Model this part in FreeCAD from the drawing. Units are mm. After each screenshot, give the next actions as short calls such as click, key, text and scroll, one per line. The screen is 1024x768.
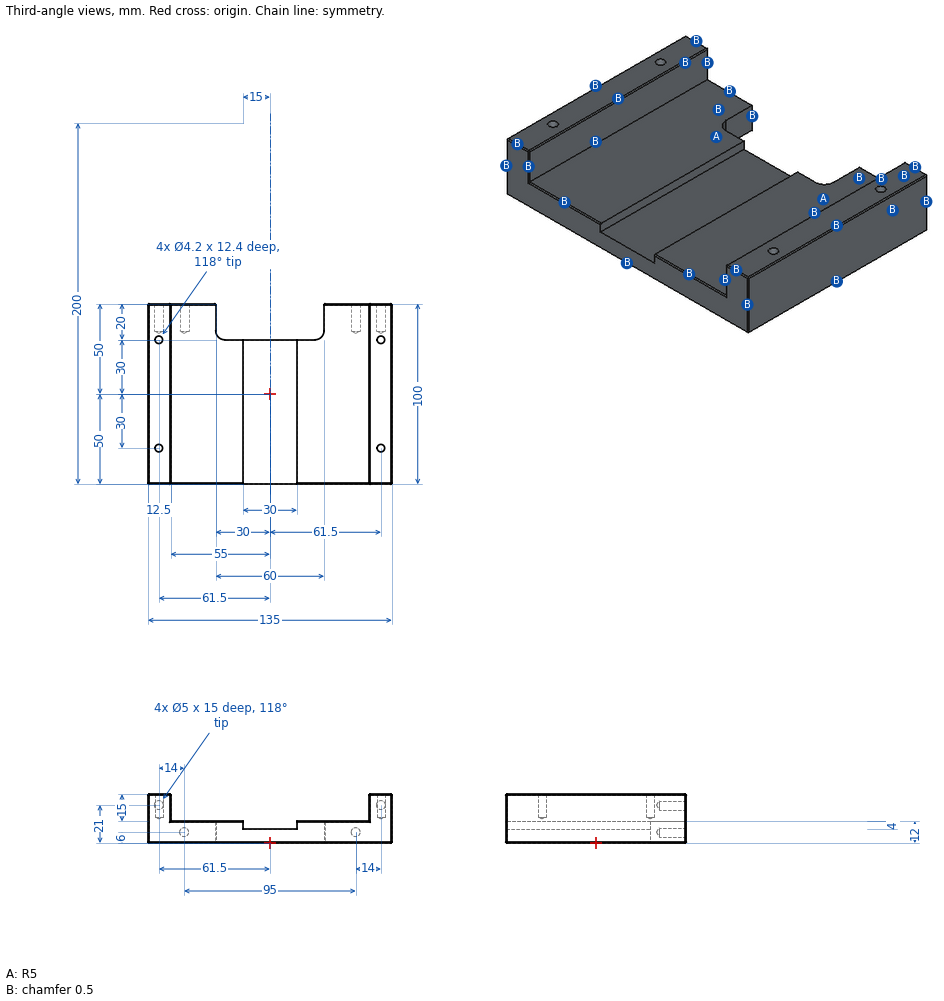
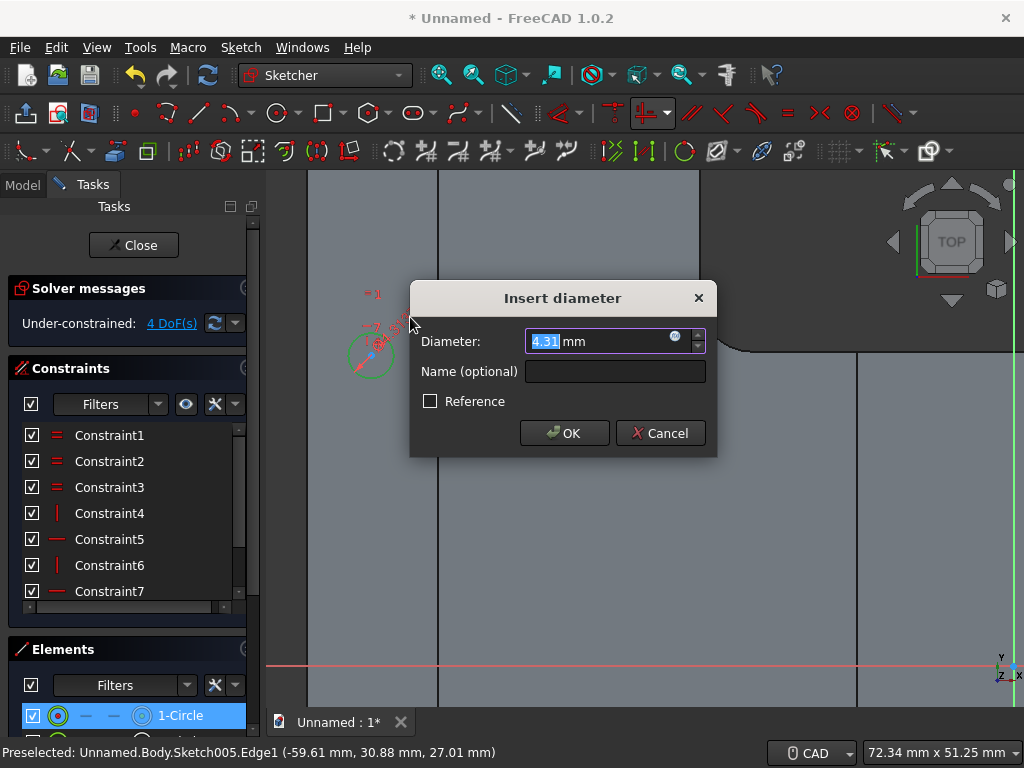
text(4.2)
key(Return)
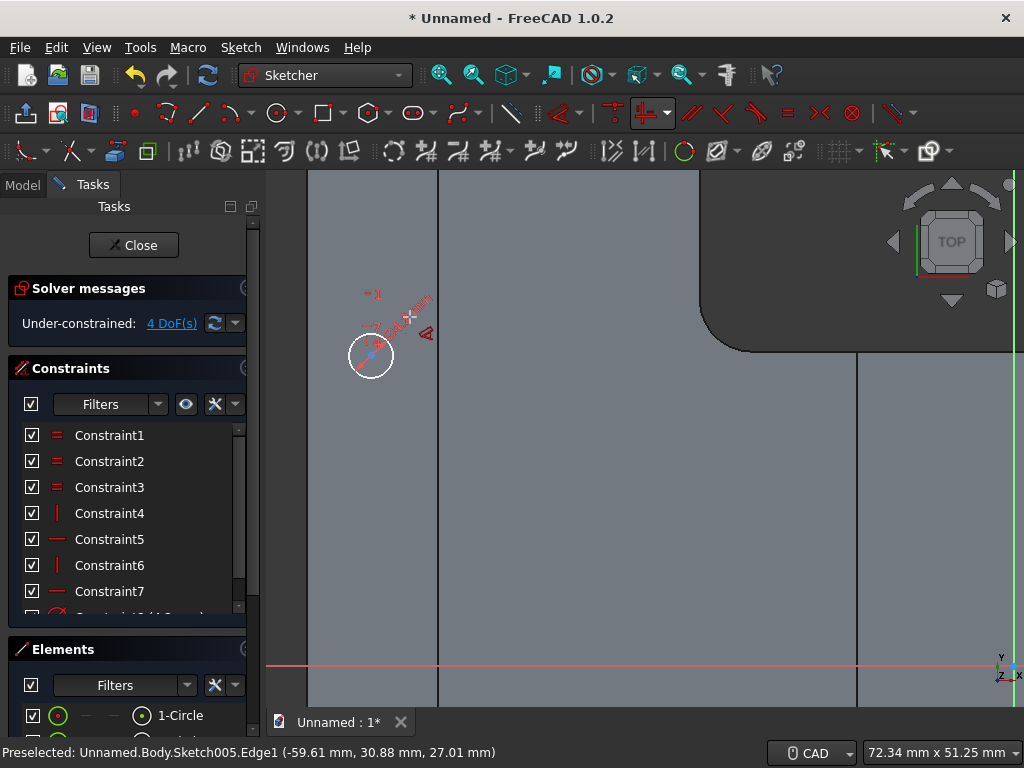
scroll(388, 340, down, 6)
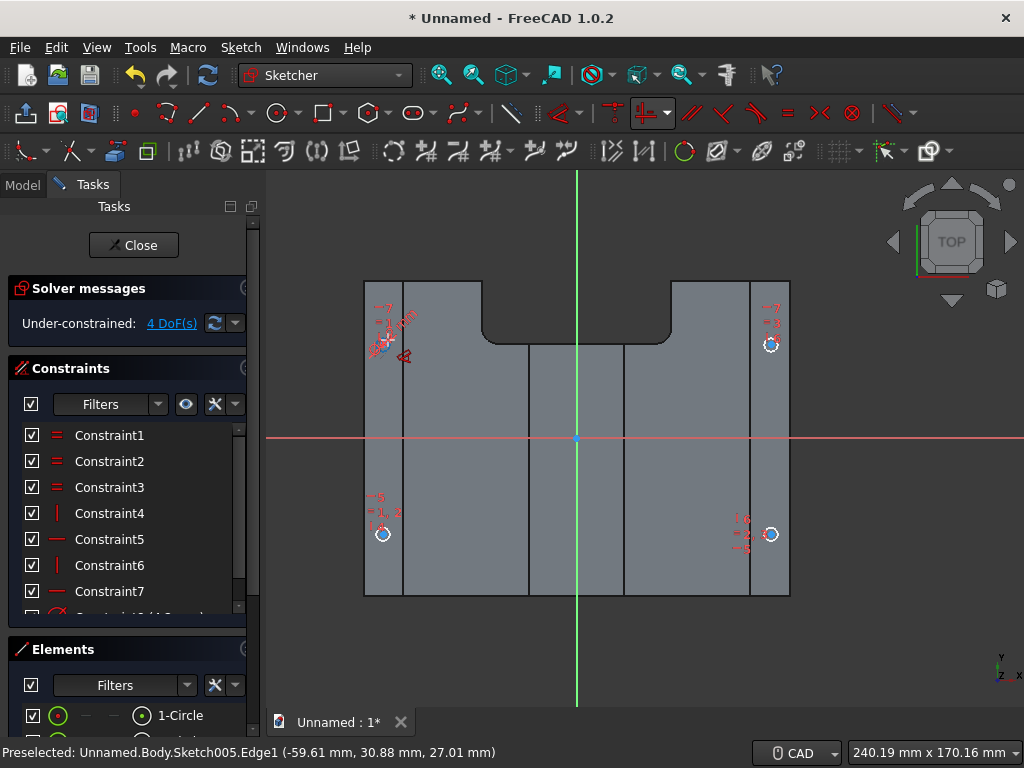
click(383, 345)
click(349, 392)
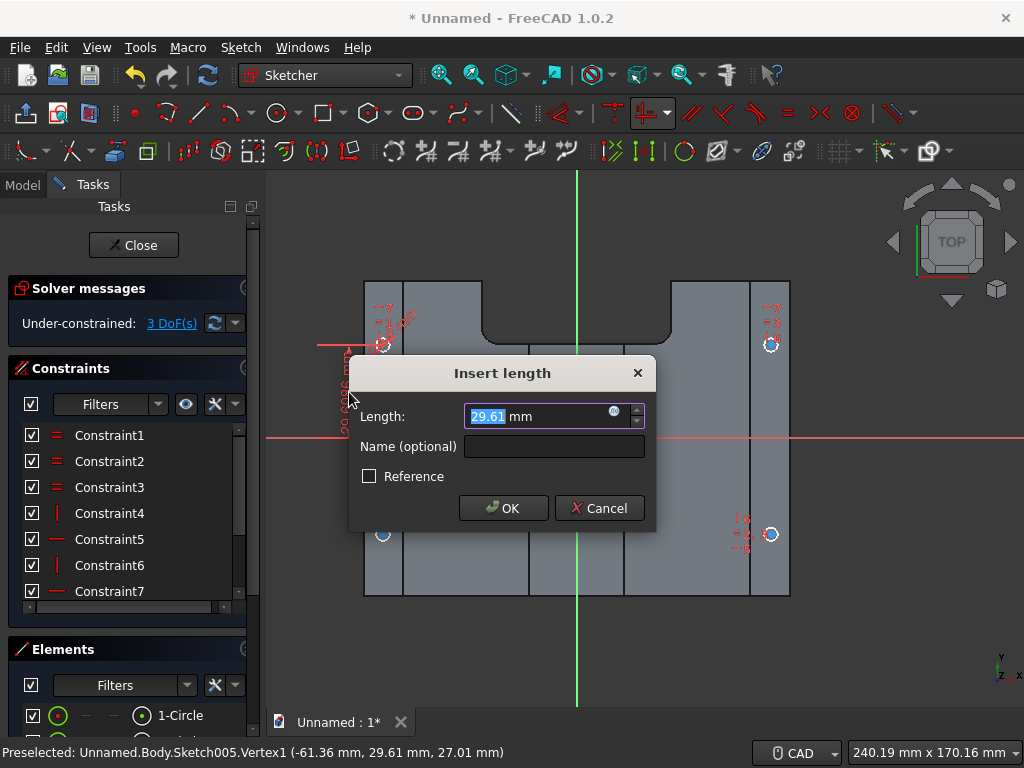
text(30)
key(Return)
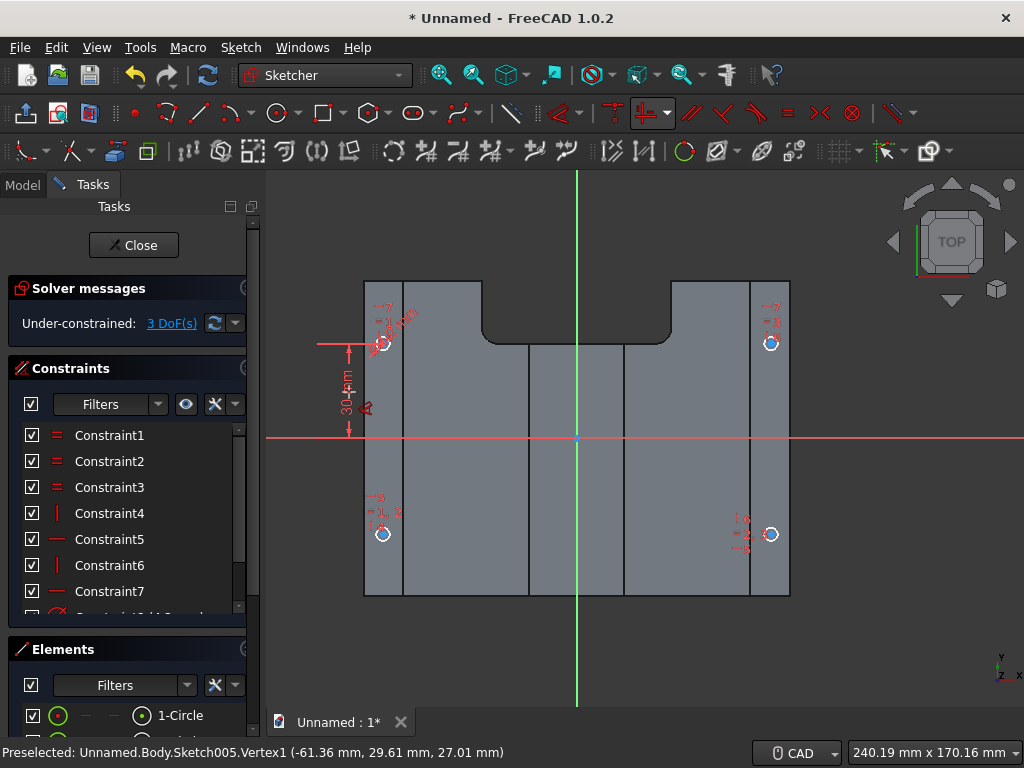
click(383, 534)
click(349, 486)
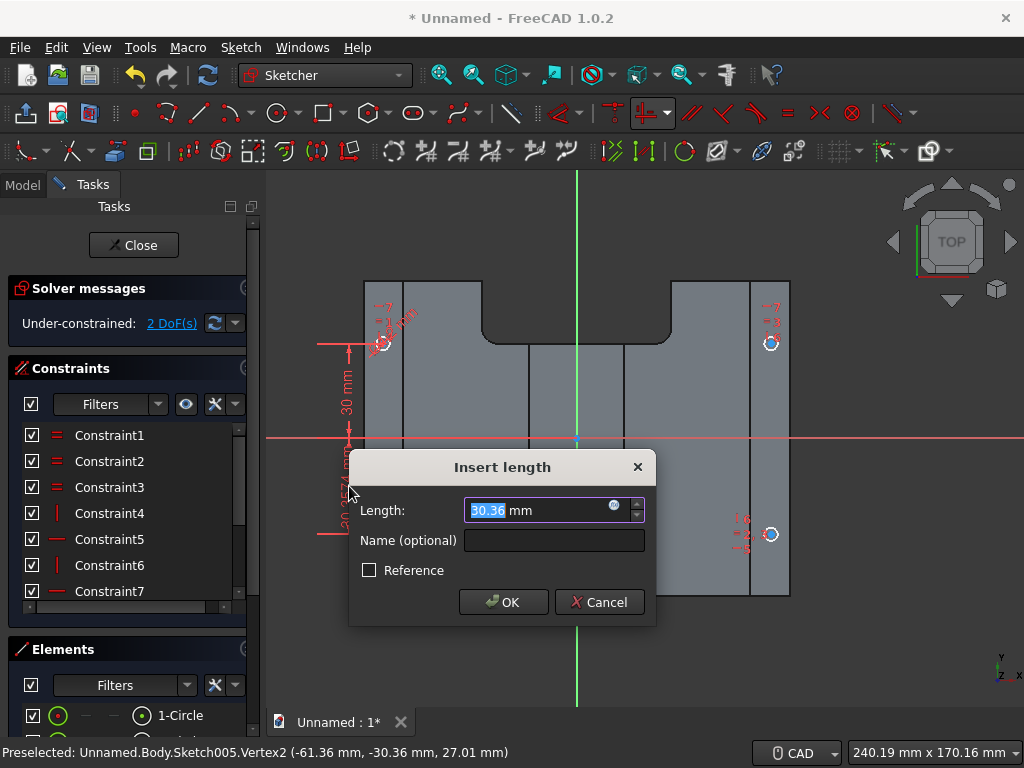
text(30)
key(Return)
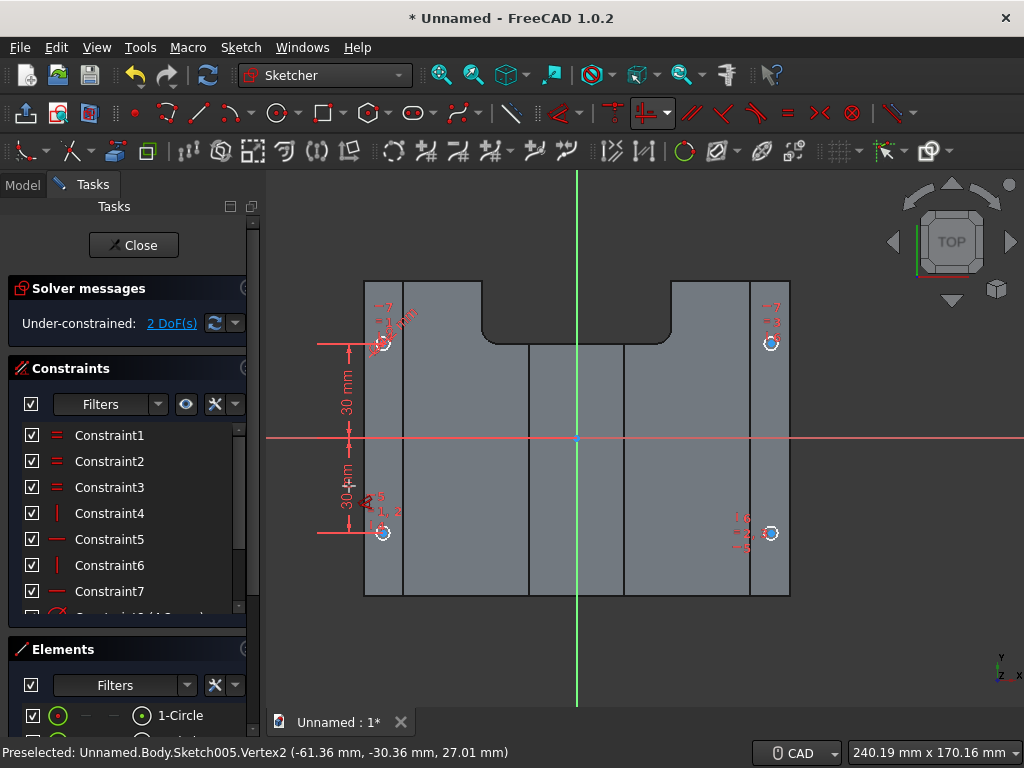
click(383, 344)
click(480, 310)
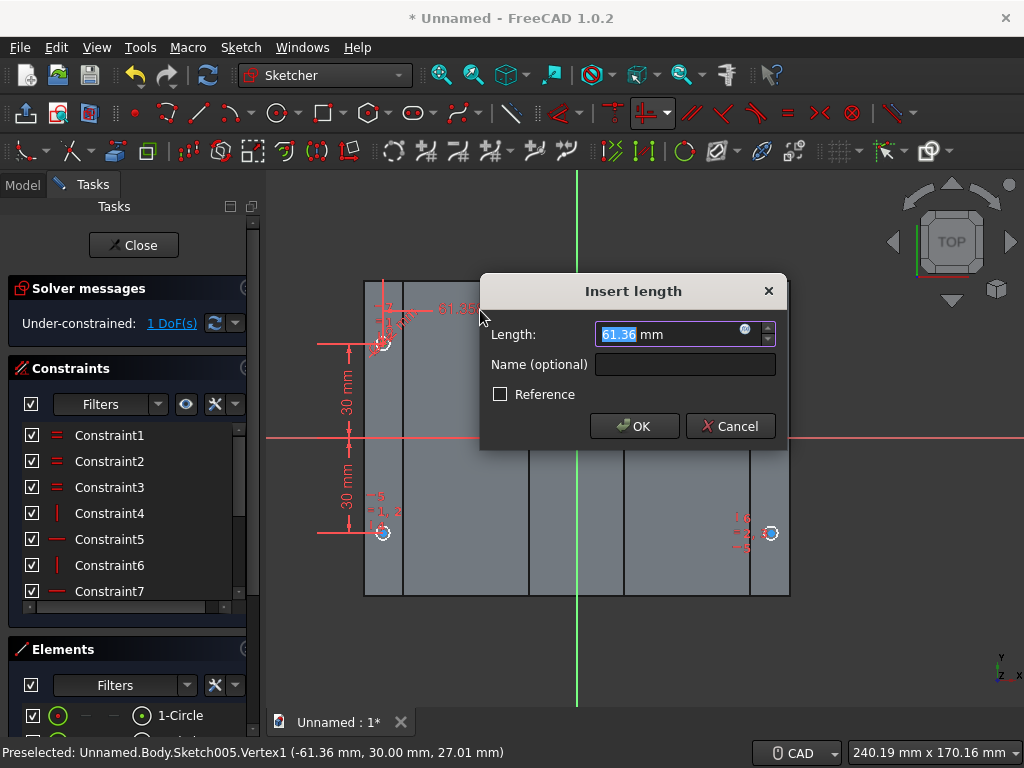
text(61.5)
key(Return)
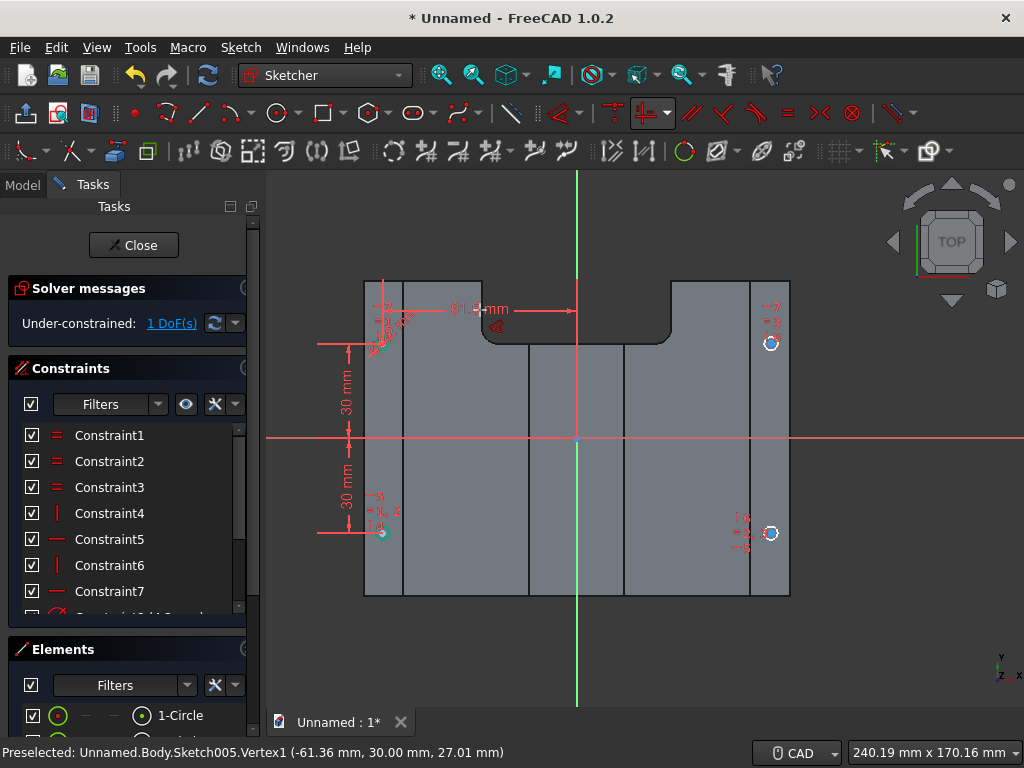
click(771, 533)
click(674, 567)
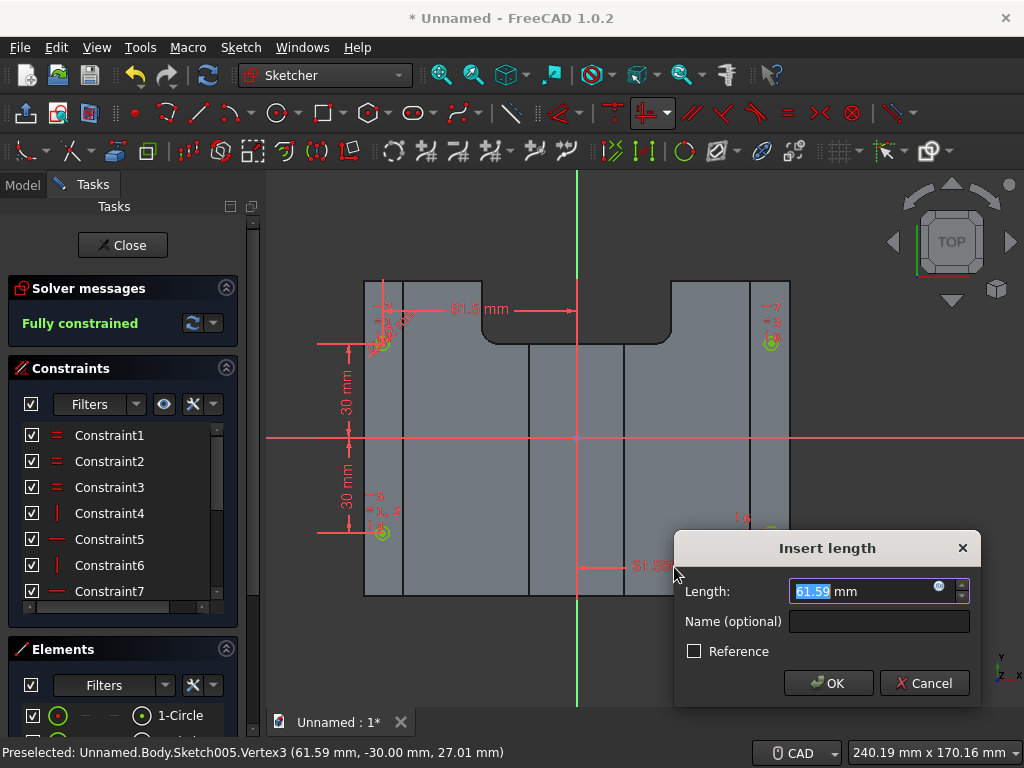
text(61.5)
key(Return)
key(Escape)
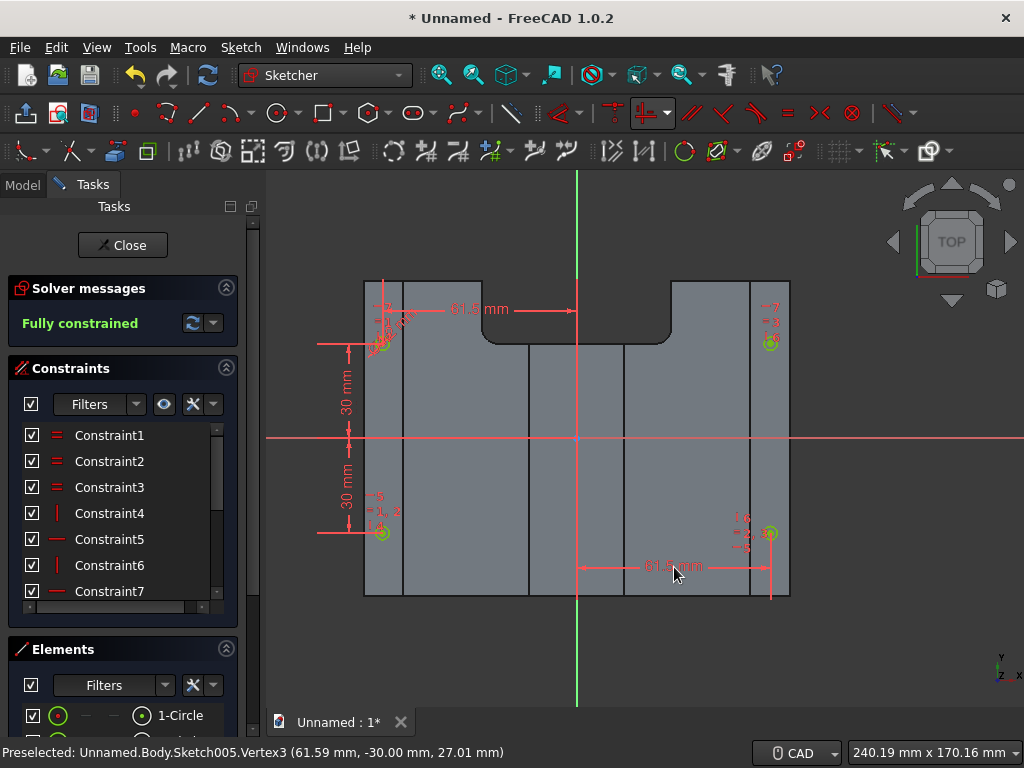
click(123, 245)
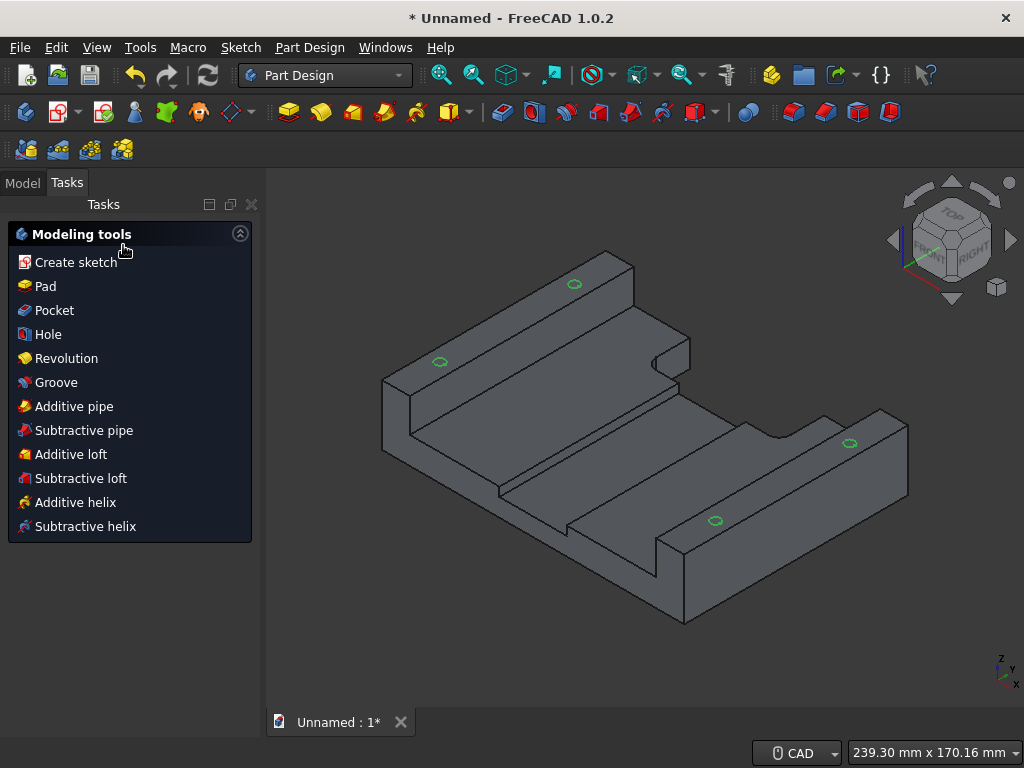
click(536, 112)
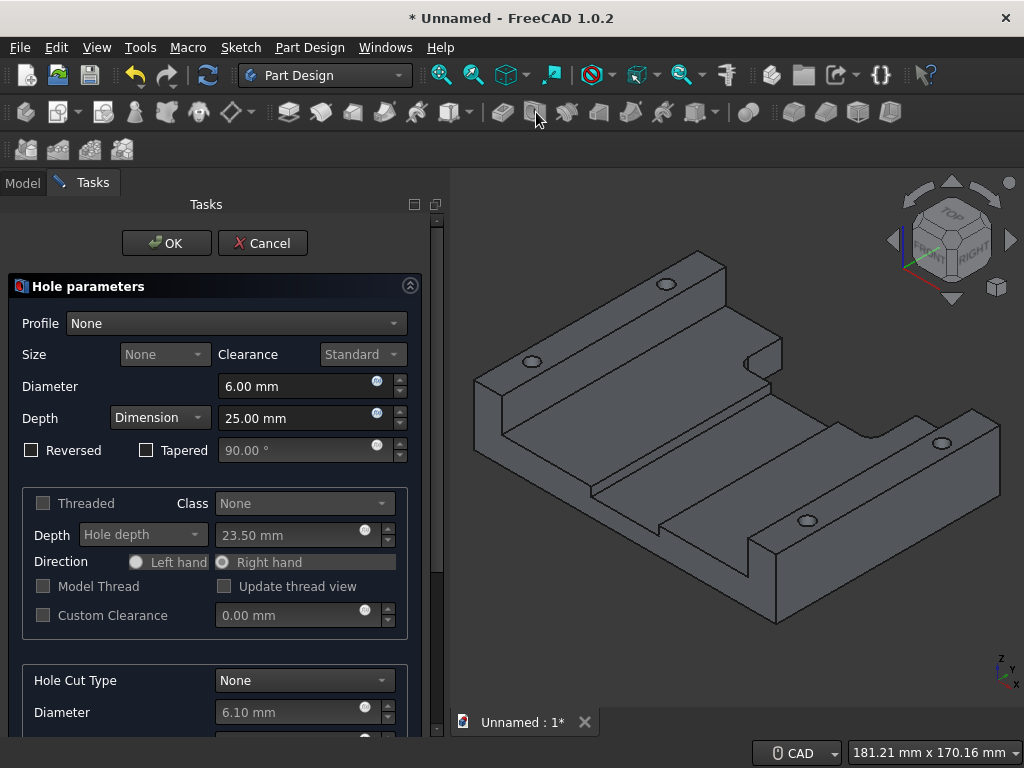
triple_click(305, 386)